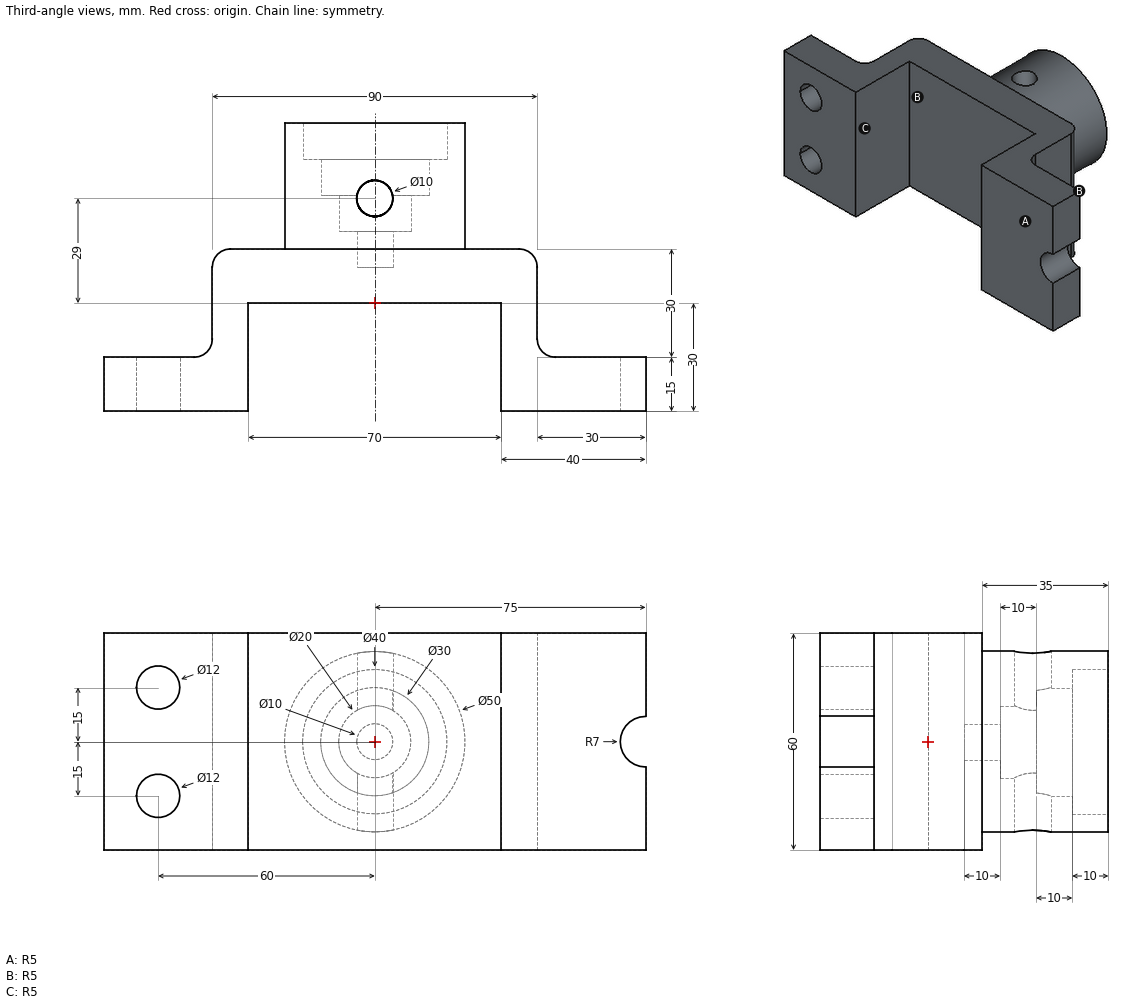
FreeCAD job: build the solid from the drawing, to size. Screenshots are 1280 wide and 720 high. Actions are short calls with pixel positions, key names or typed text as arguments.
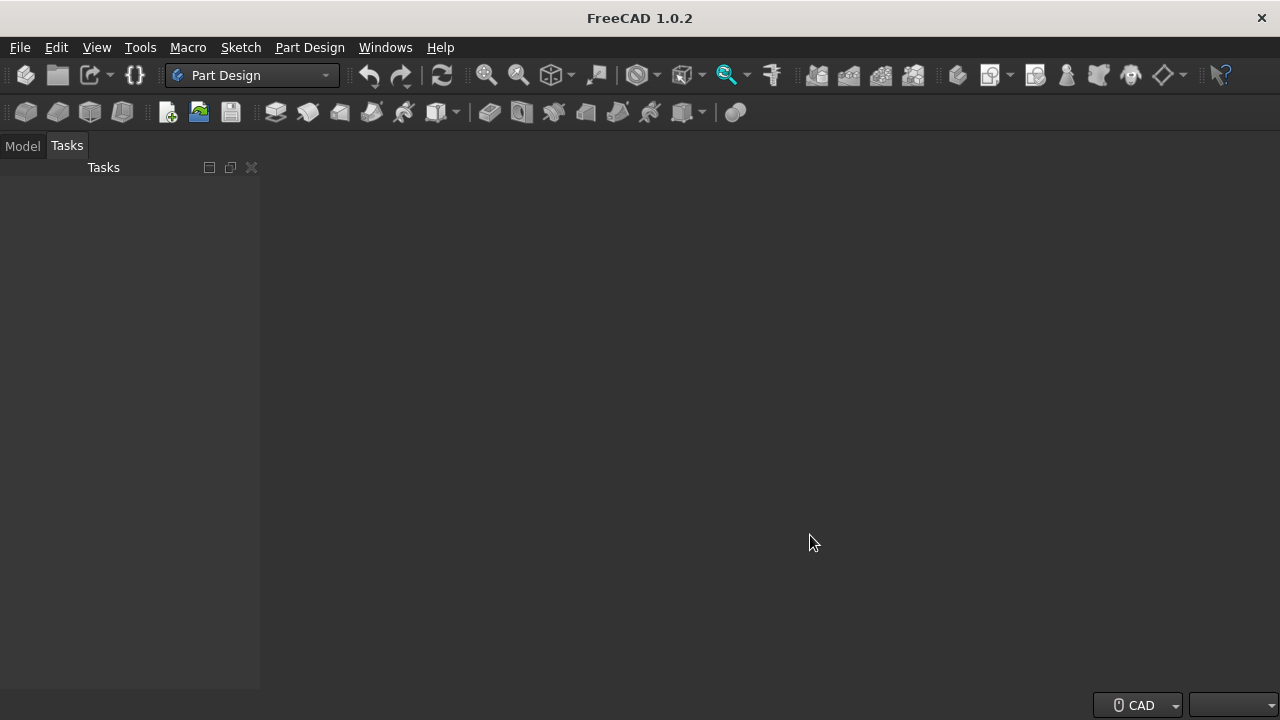
click(168, 112)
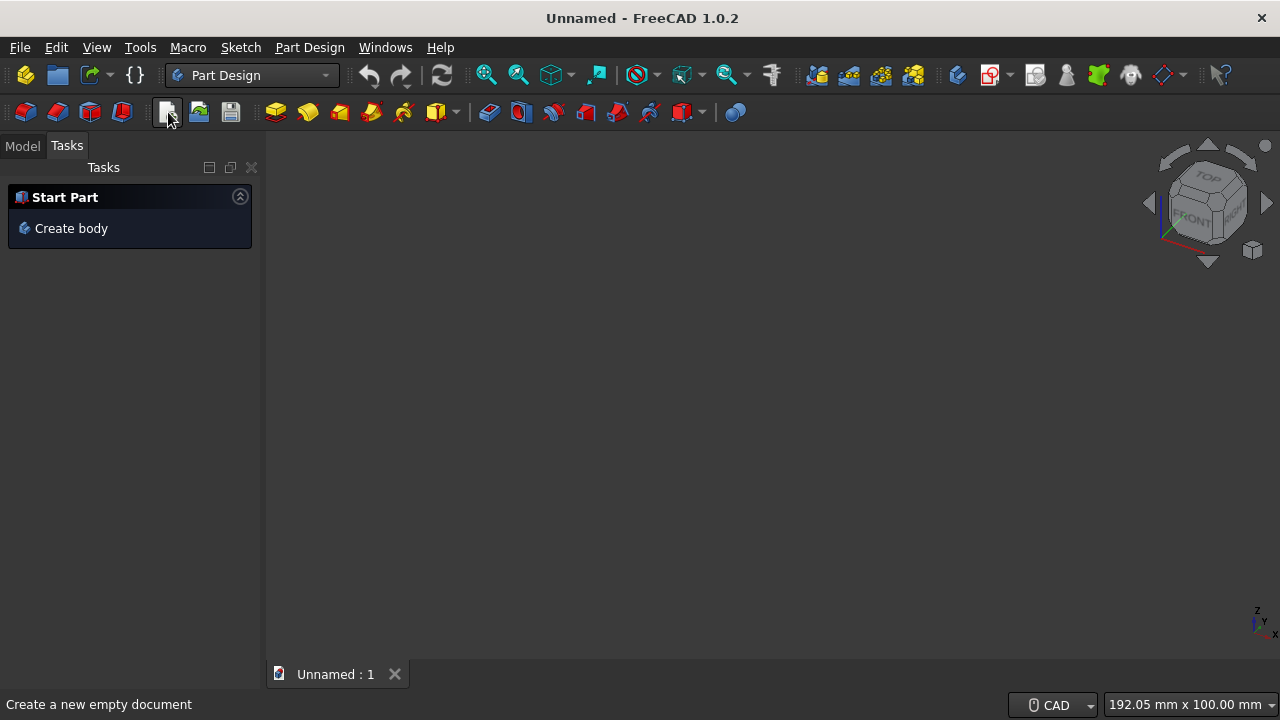
click(990, 76)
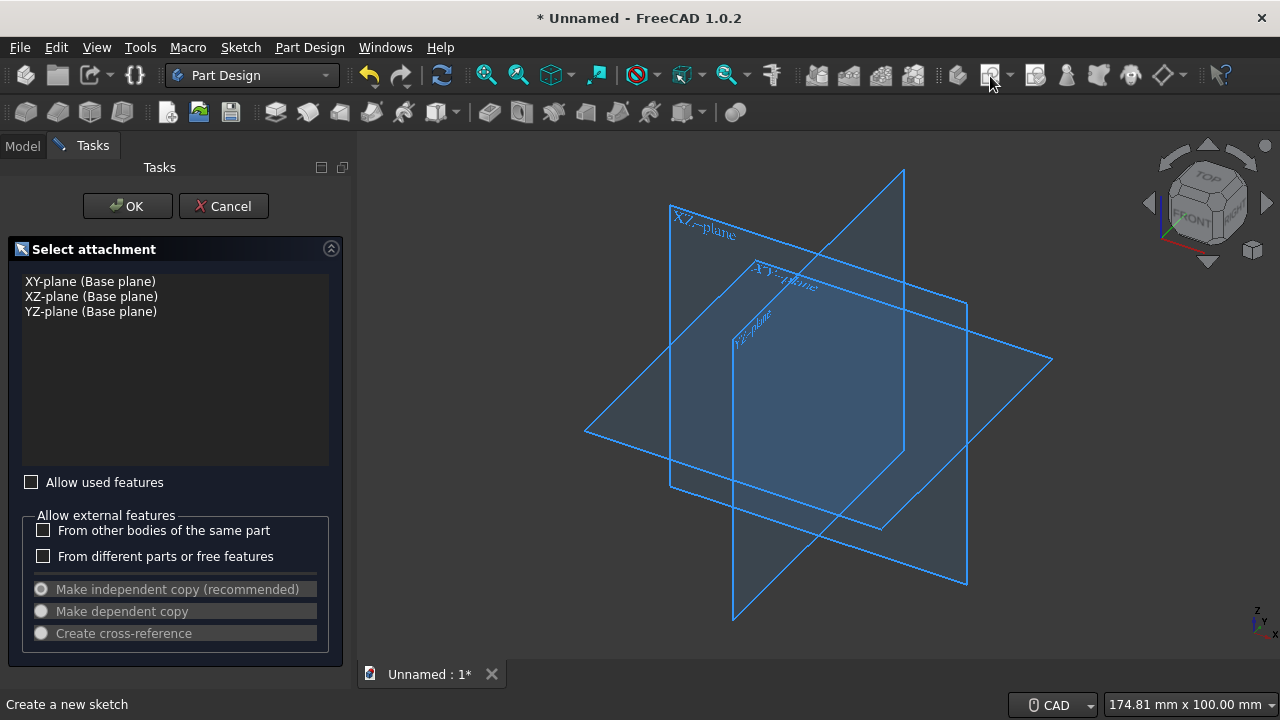
click(82, 282)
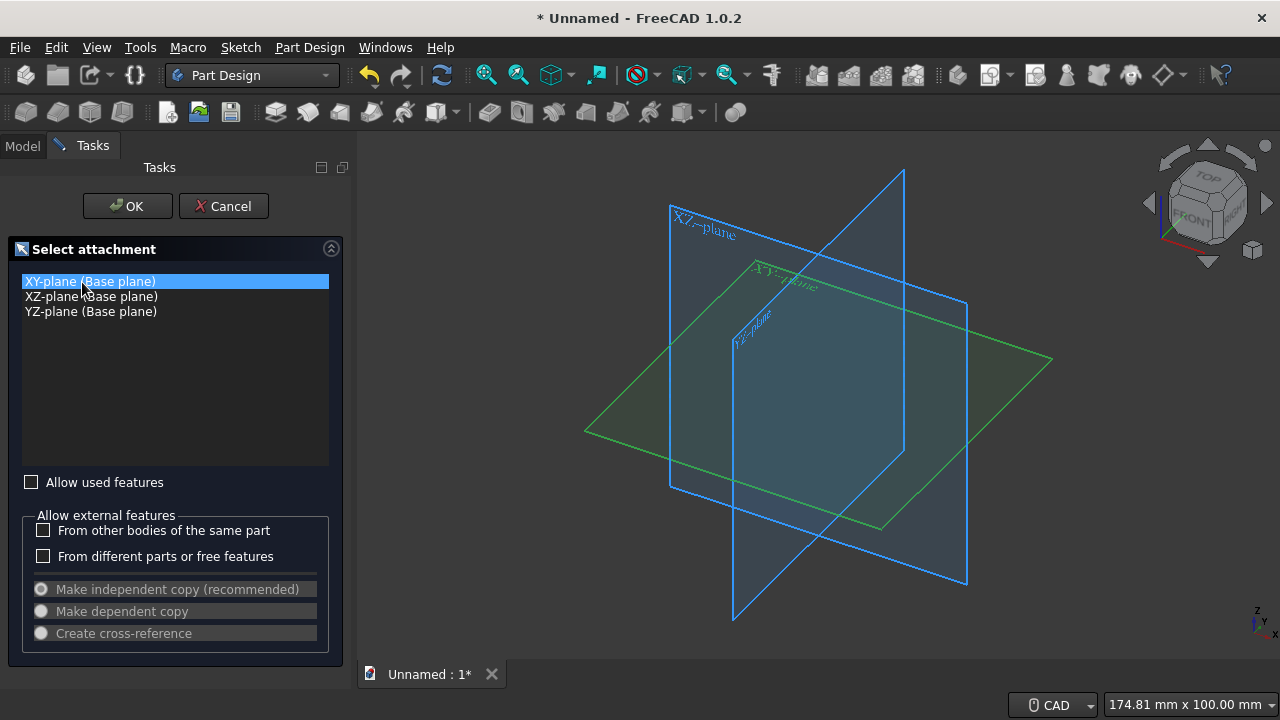
click(128, 206)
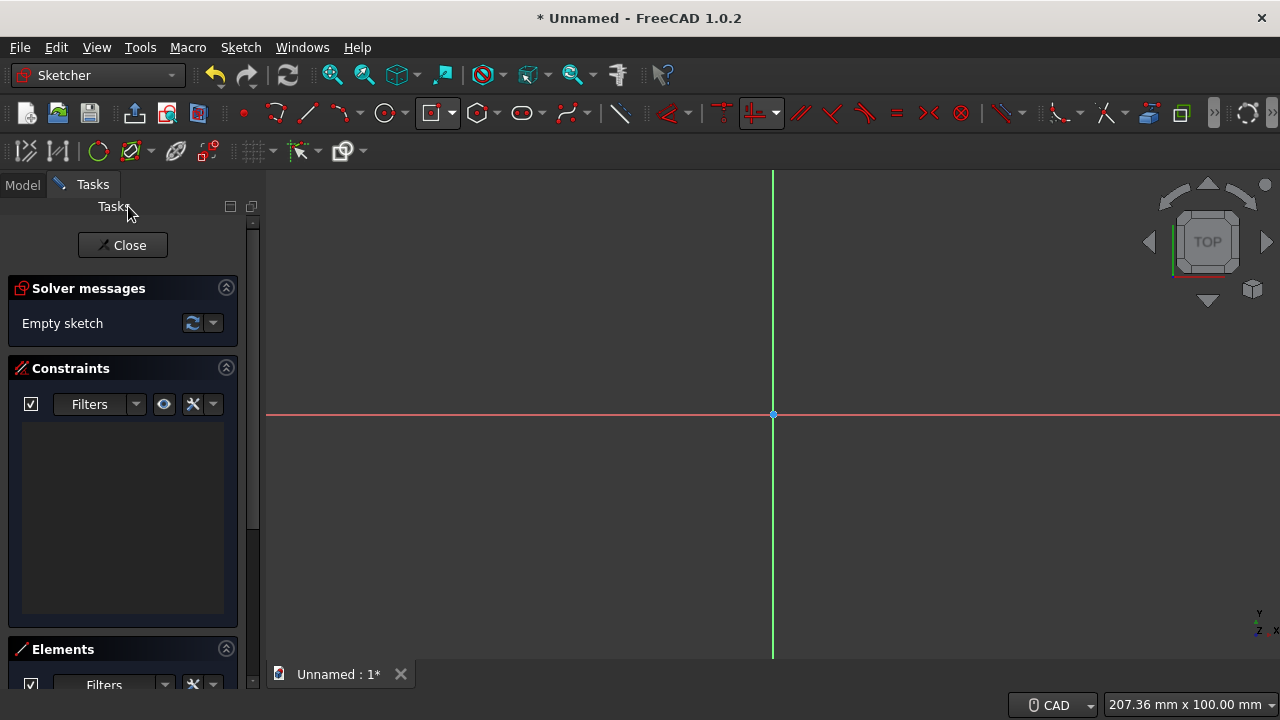
scroll(395, 249, down, 1)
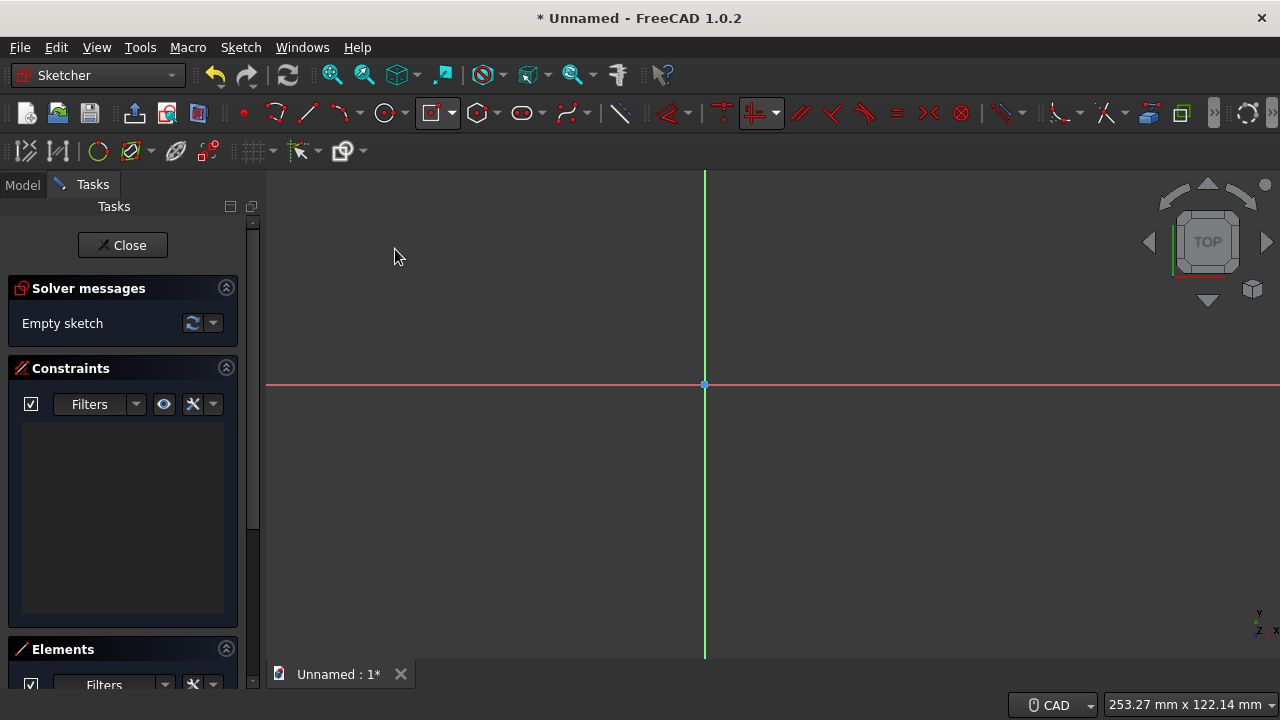
click(276, 114)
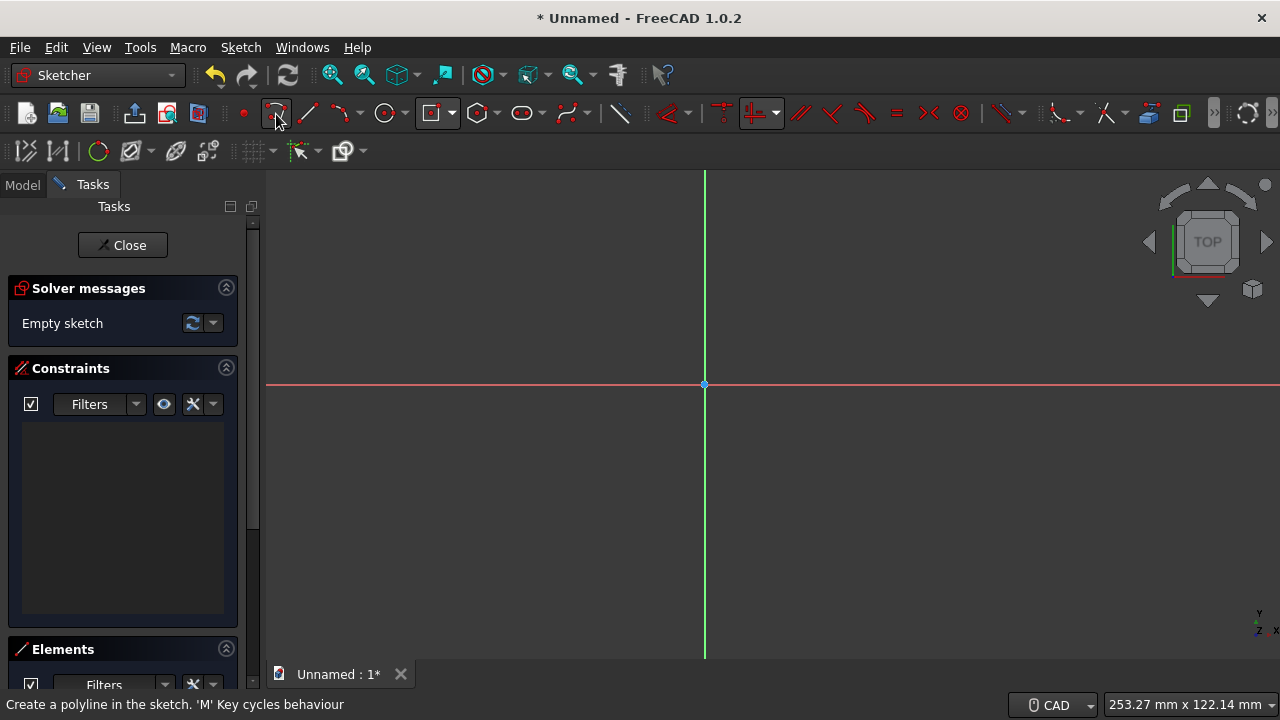
click(564, 385)
click(845, 394)
click(845, 505)
click(1005, 505)
click(1005, 445)
click(885, 445)
click(885, 324)
click(524, 324)
click(524, 445)
click(404, 445)
click(404, 505)
click(564, 505)
click(564, 385)
key(Escape)
key(Escape)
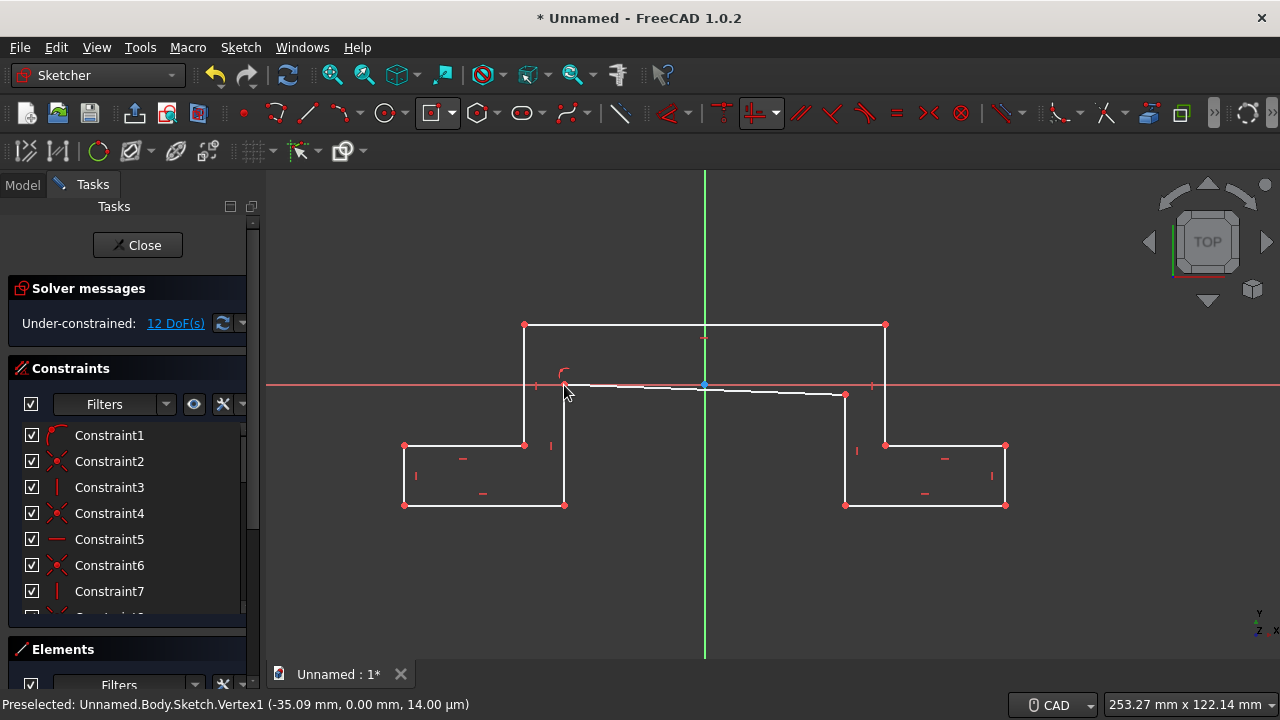
click(648, 388)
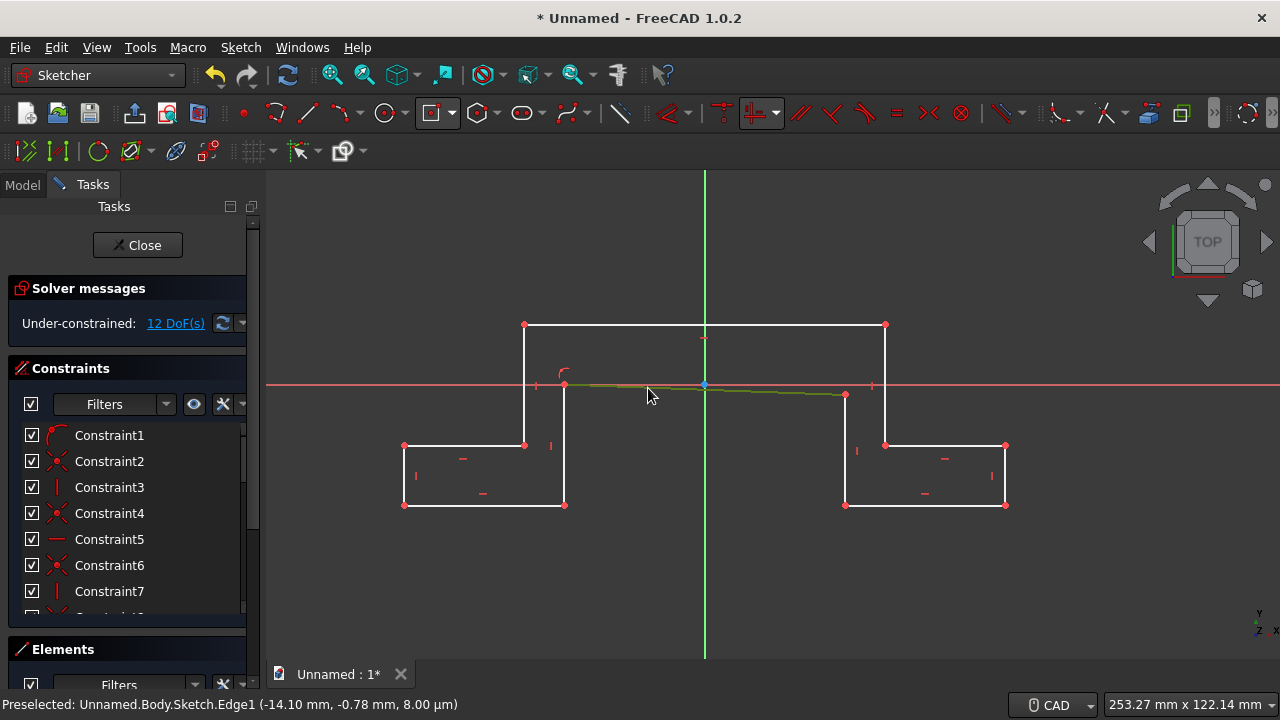
key(h)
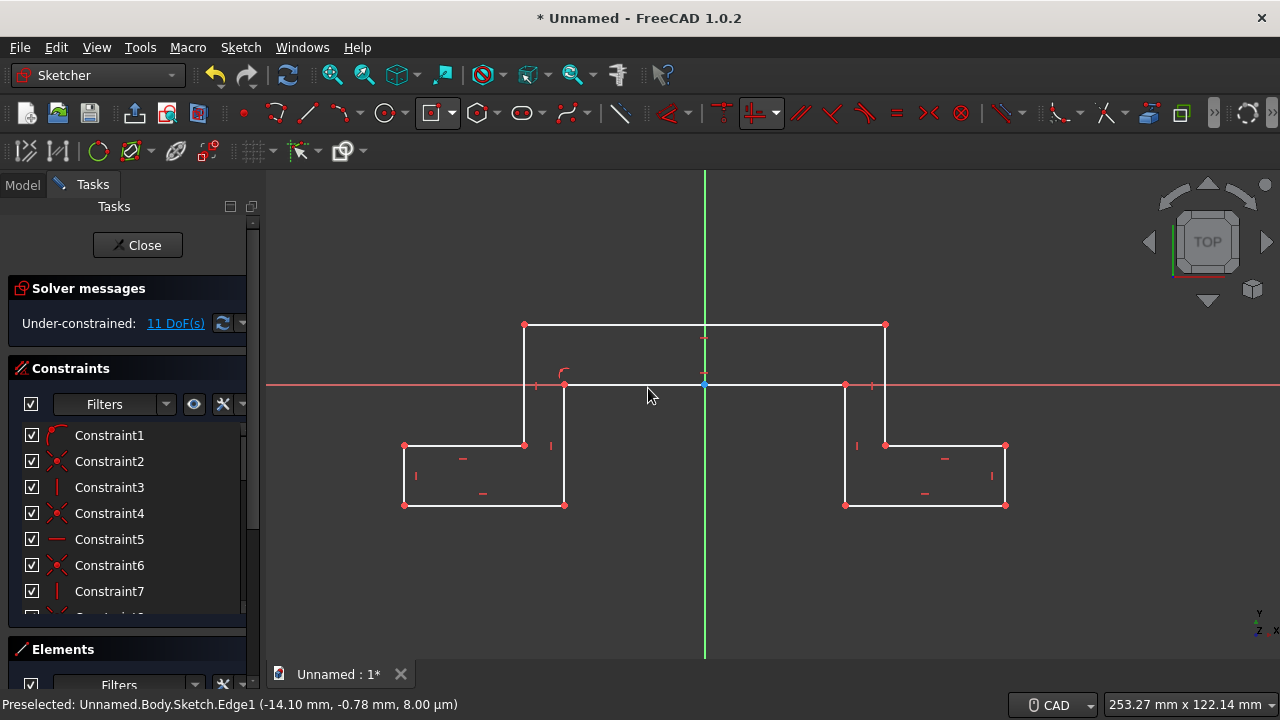
click(885, 446)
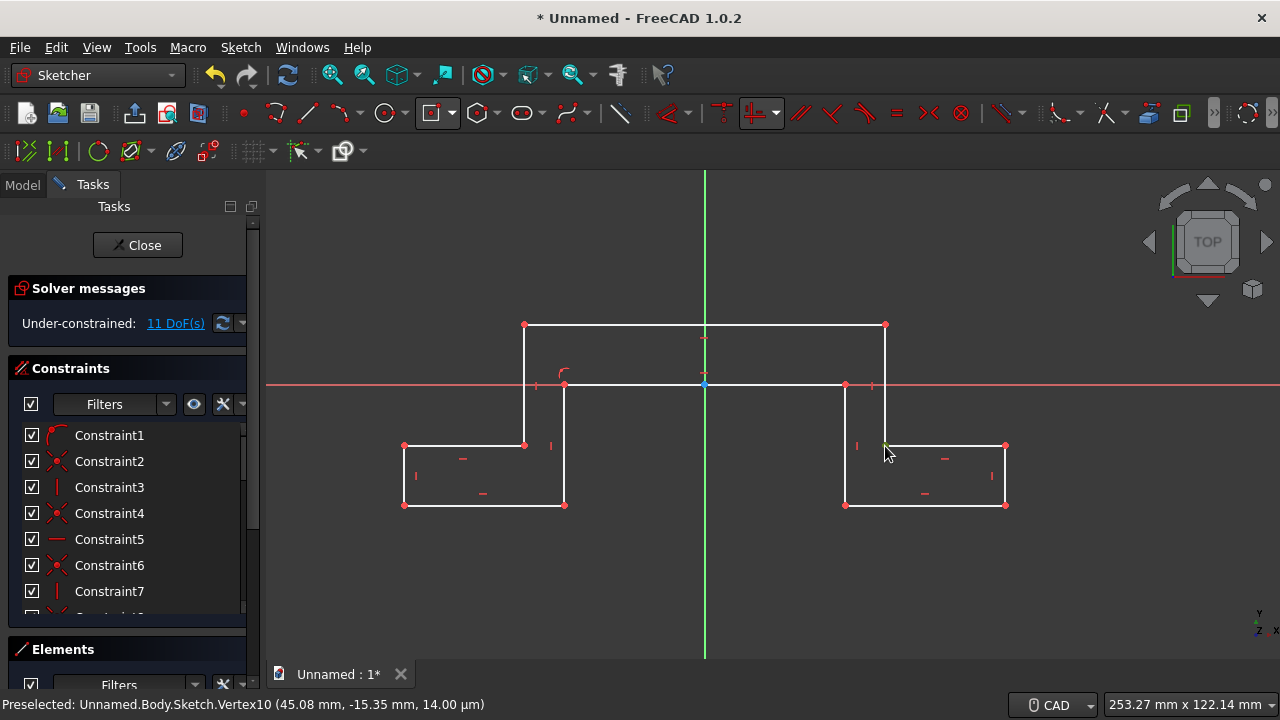
click(524, 446)